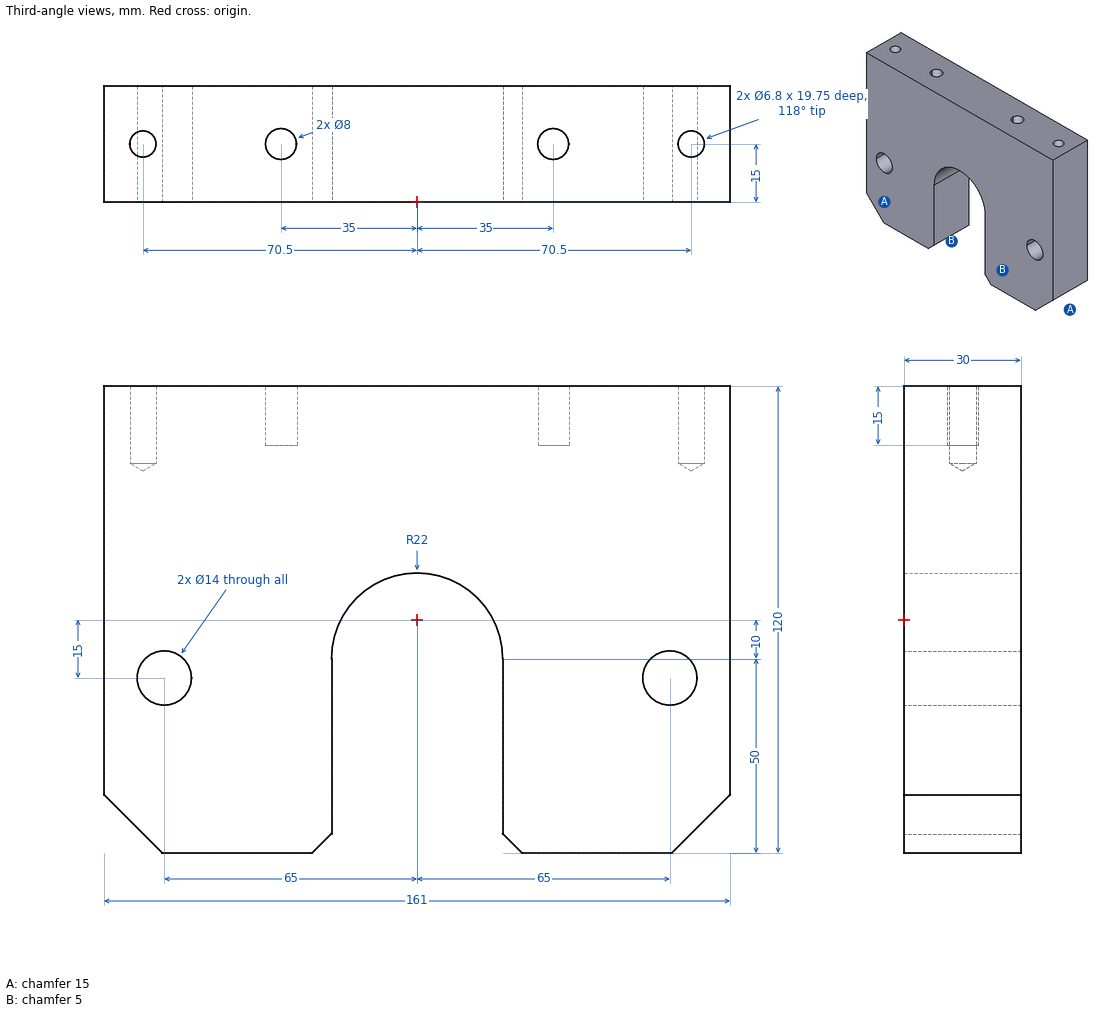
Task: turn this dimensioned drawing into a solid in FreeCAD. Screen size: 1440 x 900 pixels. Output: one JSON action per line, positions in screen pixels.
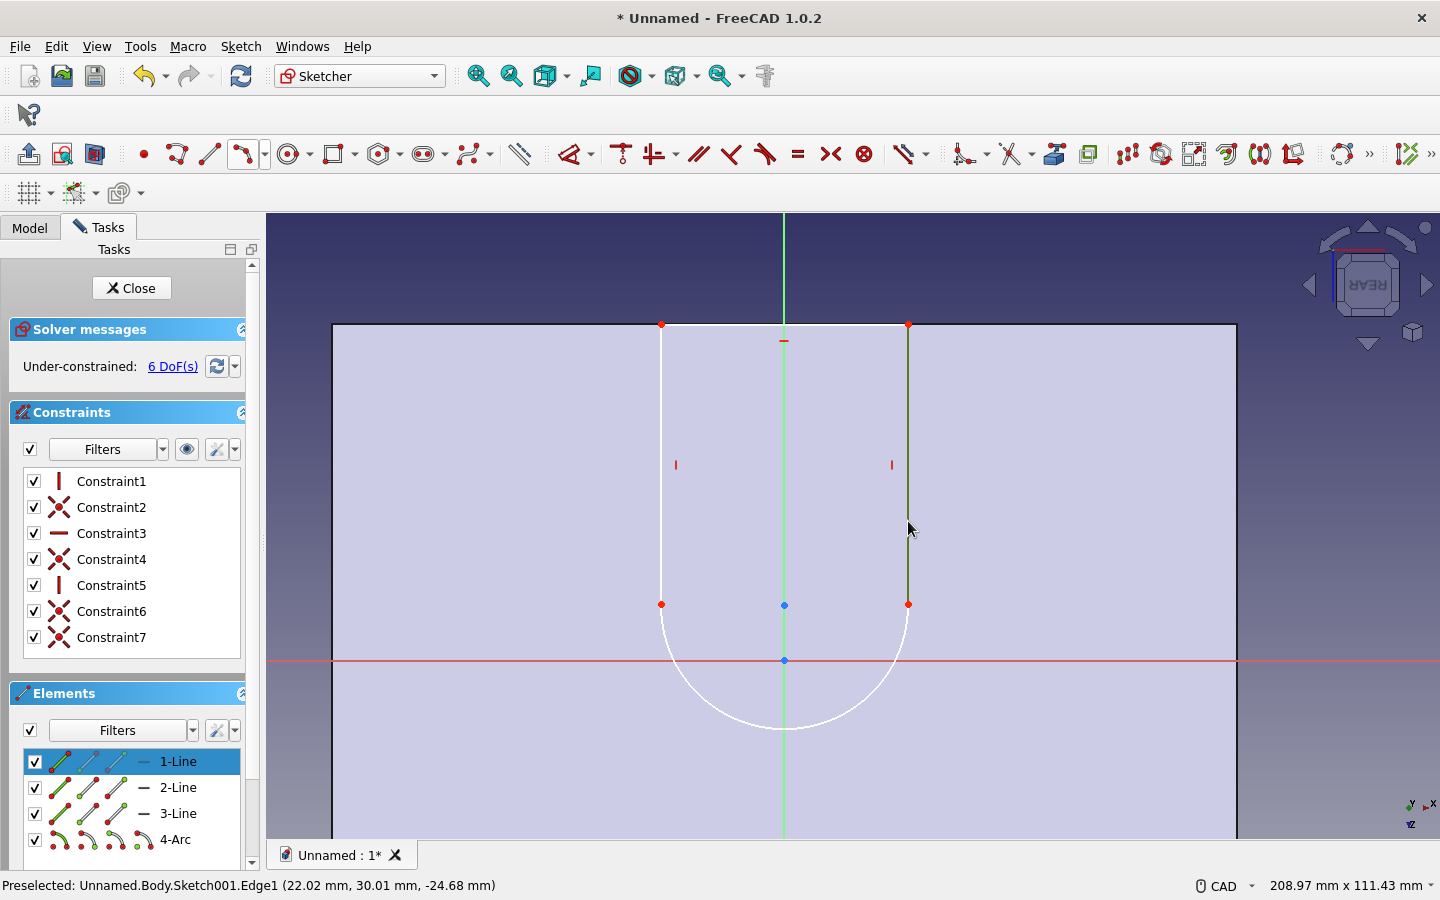
{"action": "left_click", "coordinate": [712, 705]}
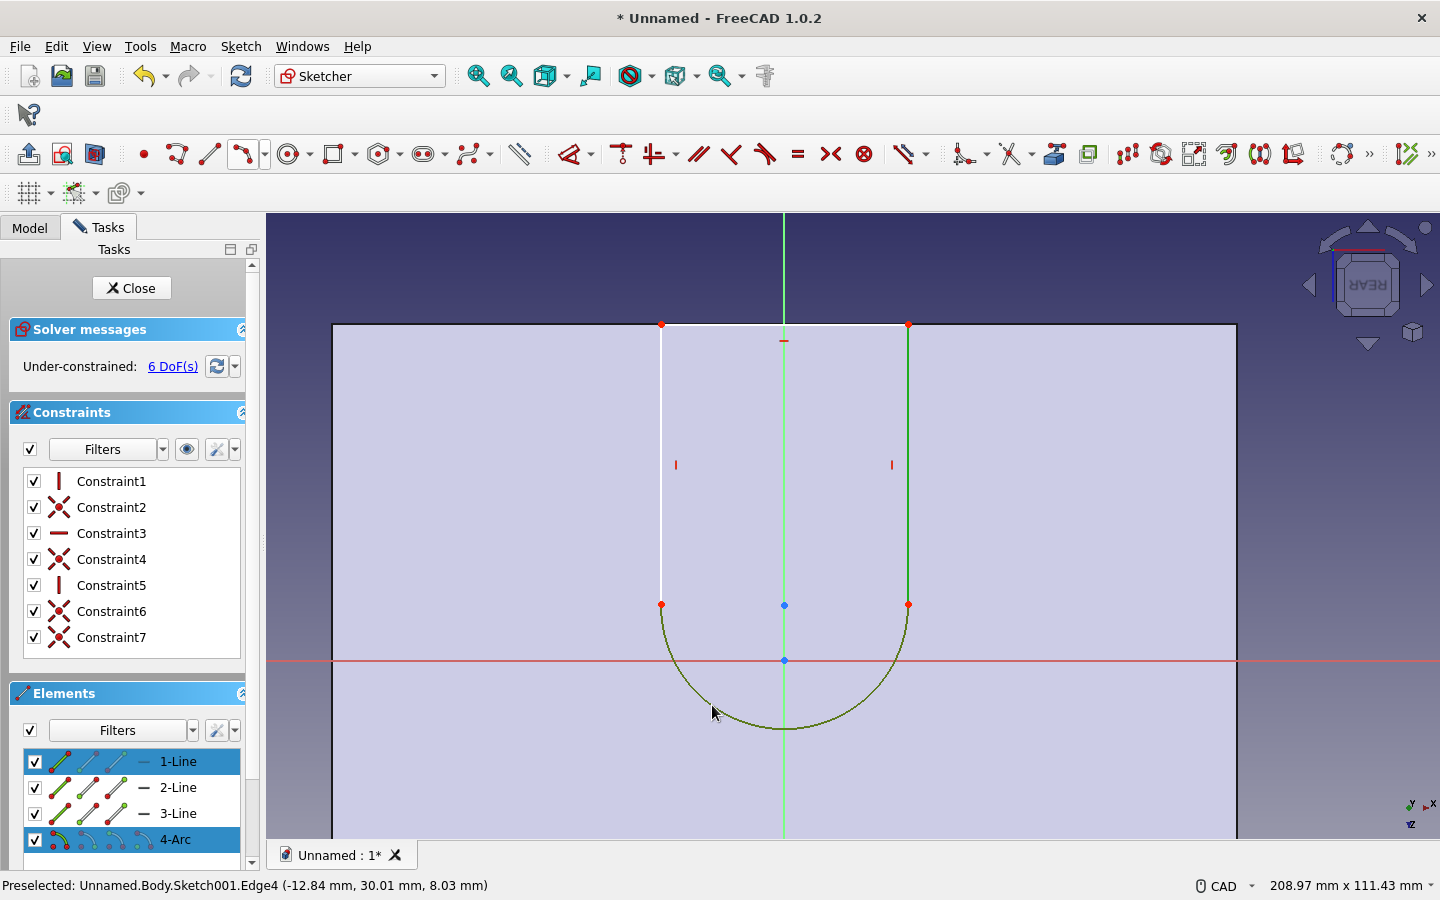
{"action": "key", "text": "t"}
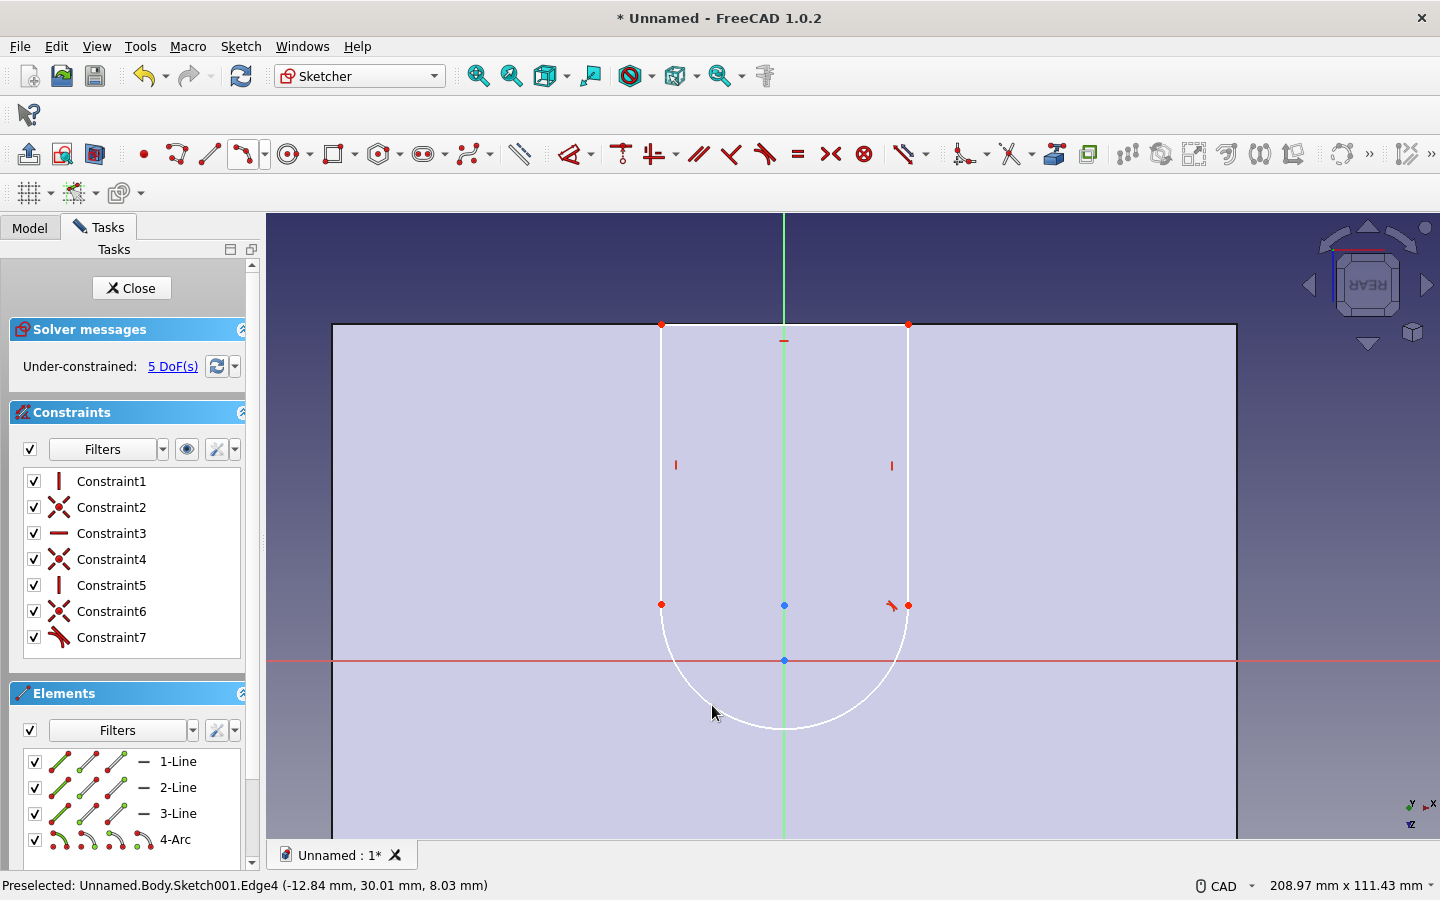
{"action": "left_click", "coordinate": [661, 409]}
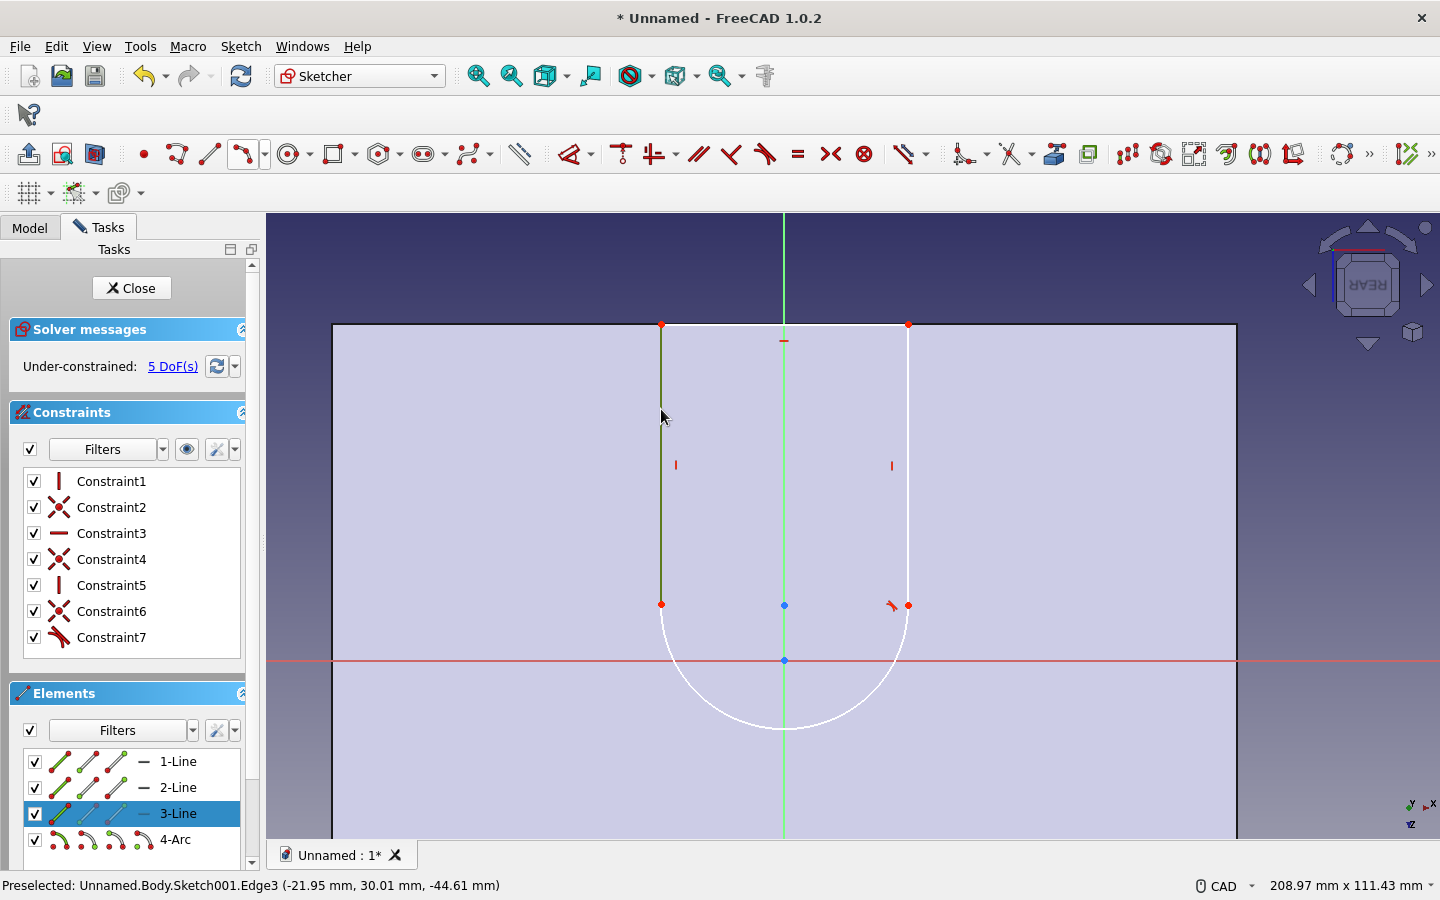
{"action": "left_click", "coordinate": [712, 705]}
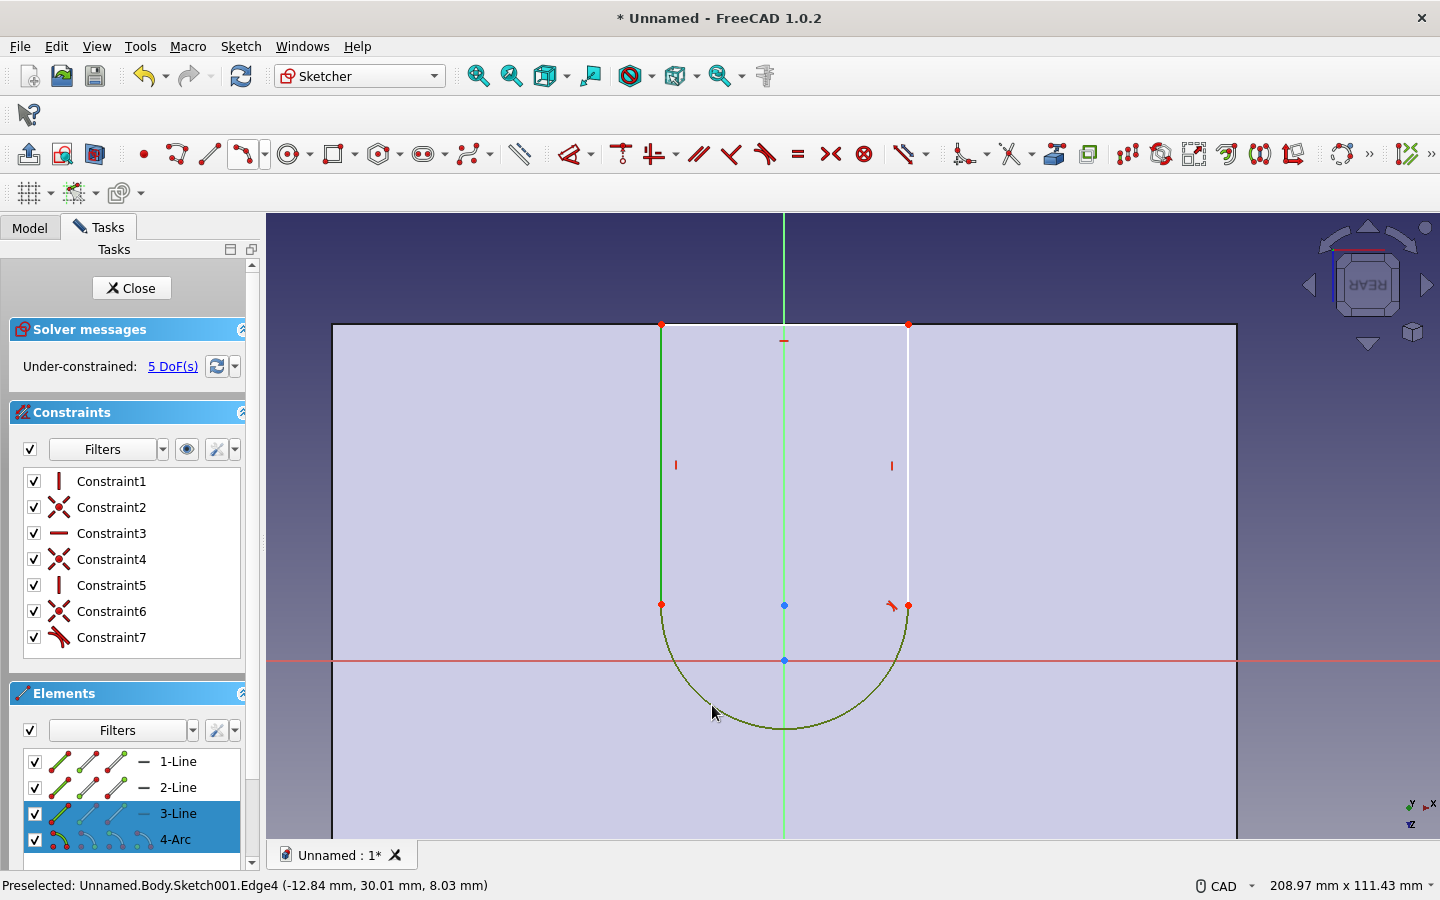
{"action": "left_click", "coordinate": [765, 154]}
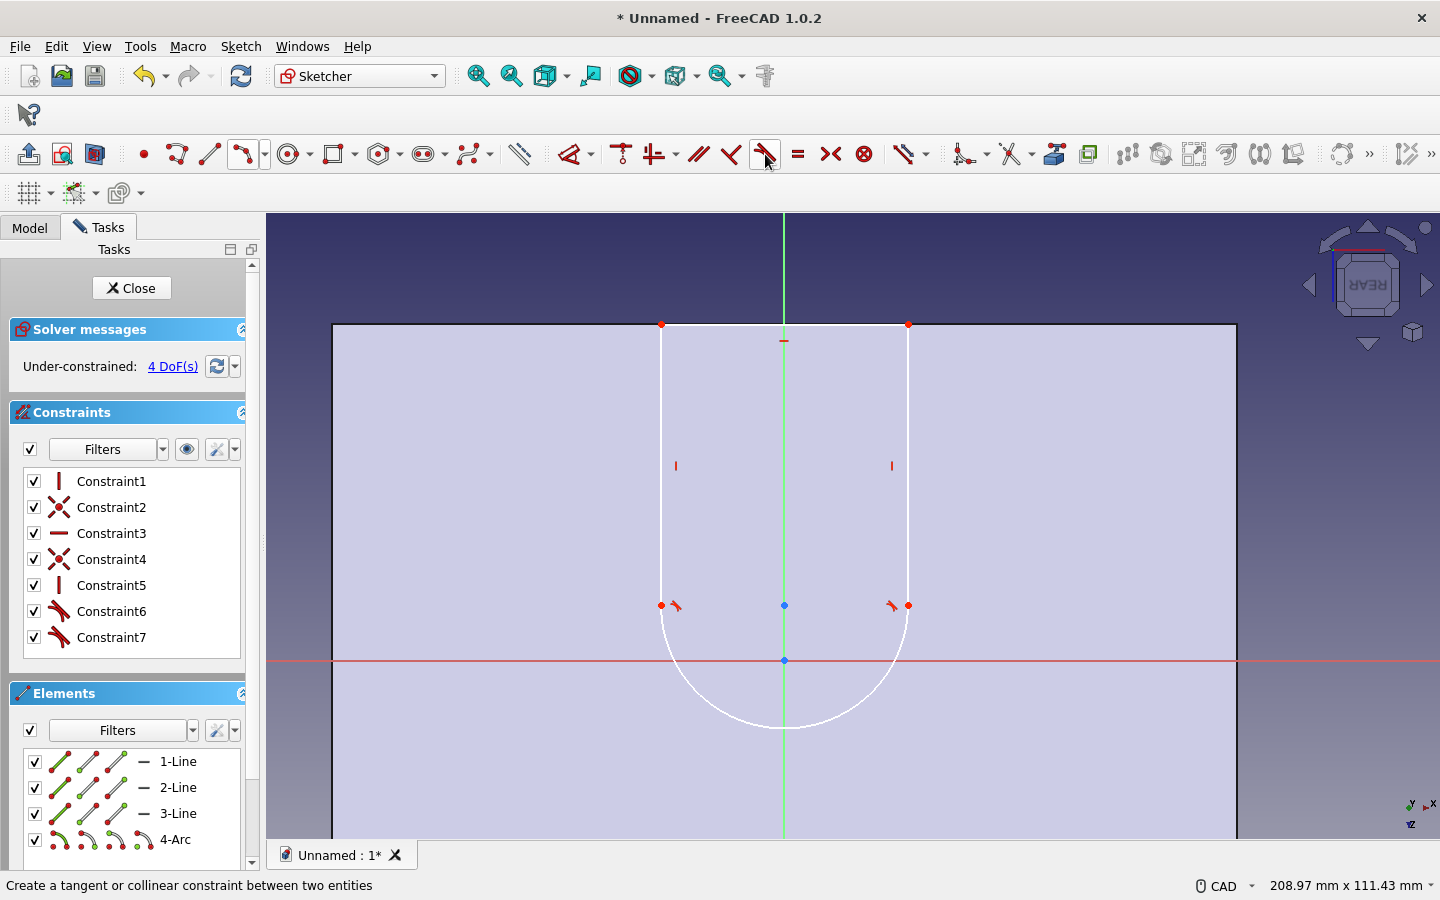
{"action": "left_click", "coordinate": [784, 605]}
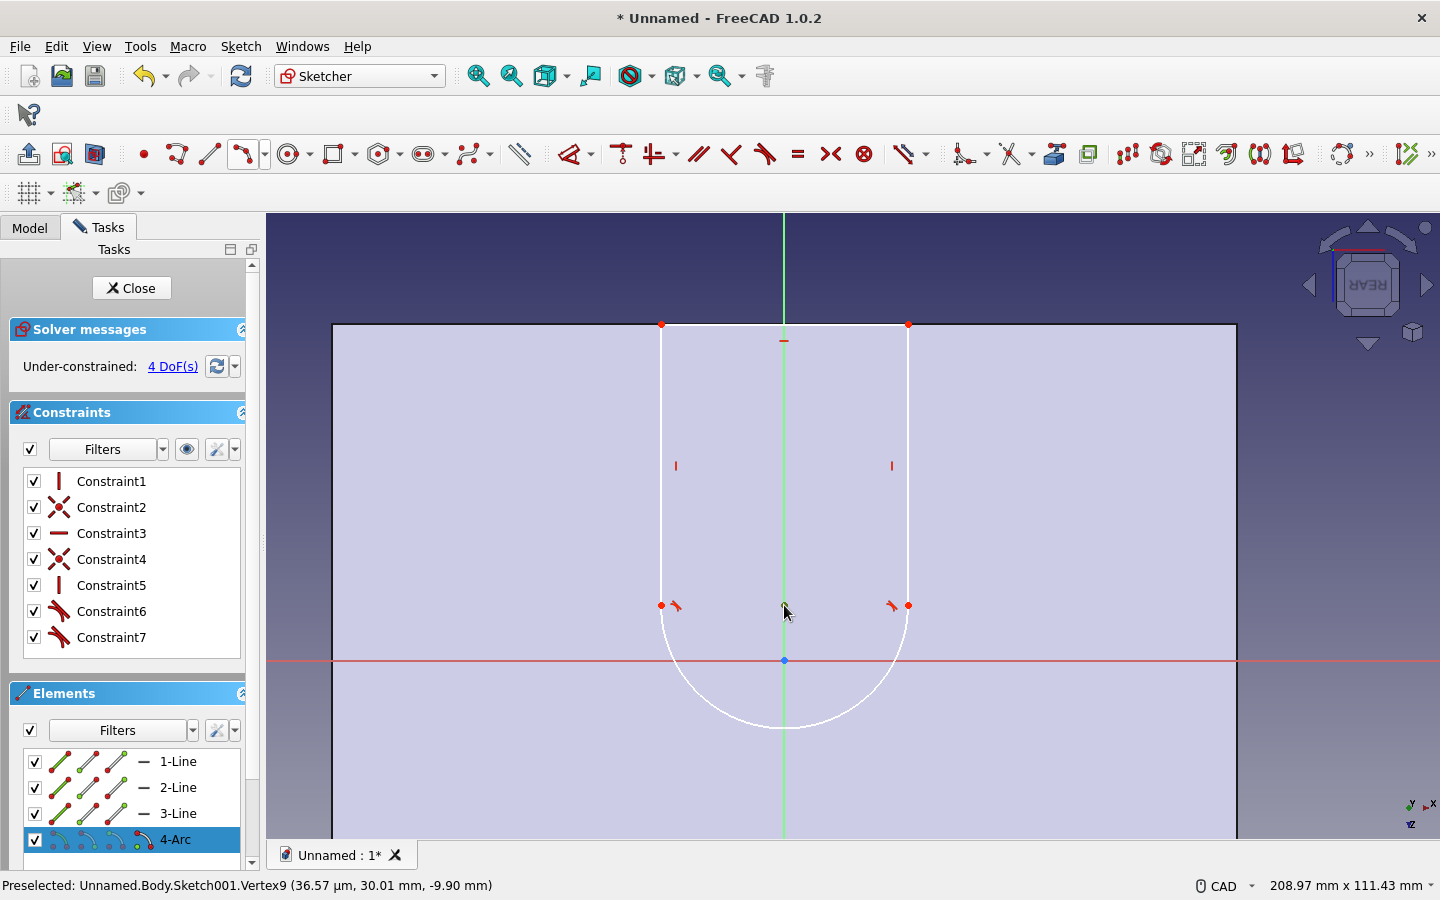
{"action": "left_click", "coordinate": [784, 770]}